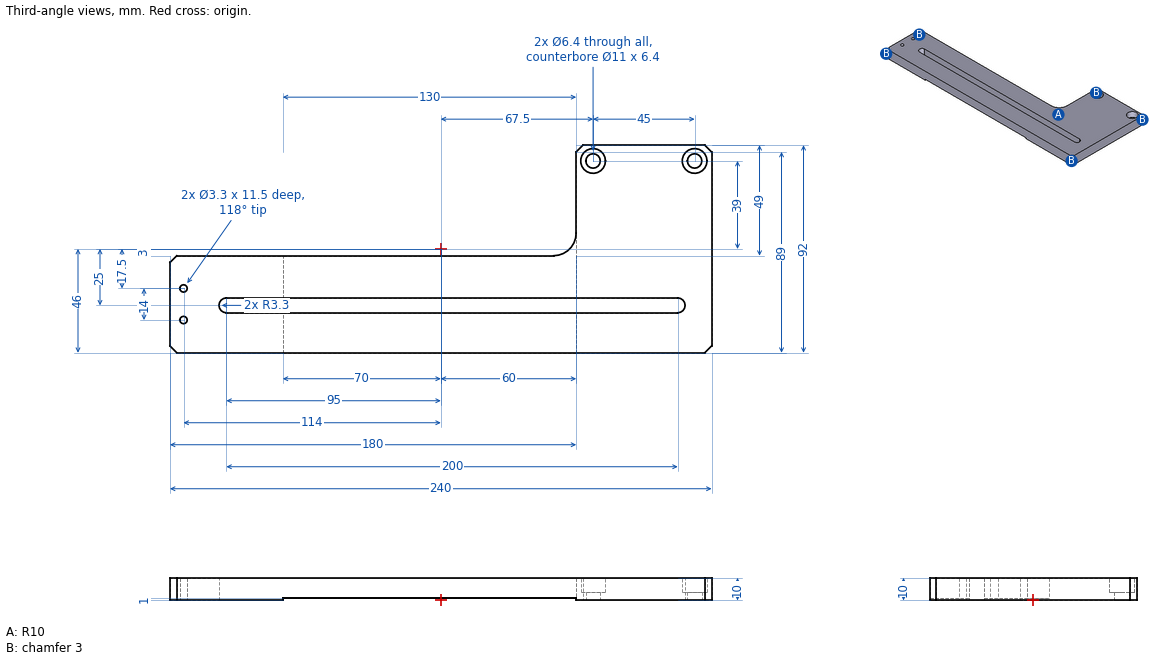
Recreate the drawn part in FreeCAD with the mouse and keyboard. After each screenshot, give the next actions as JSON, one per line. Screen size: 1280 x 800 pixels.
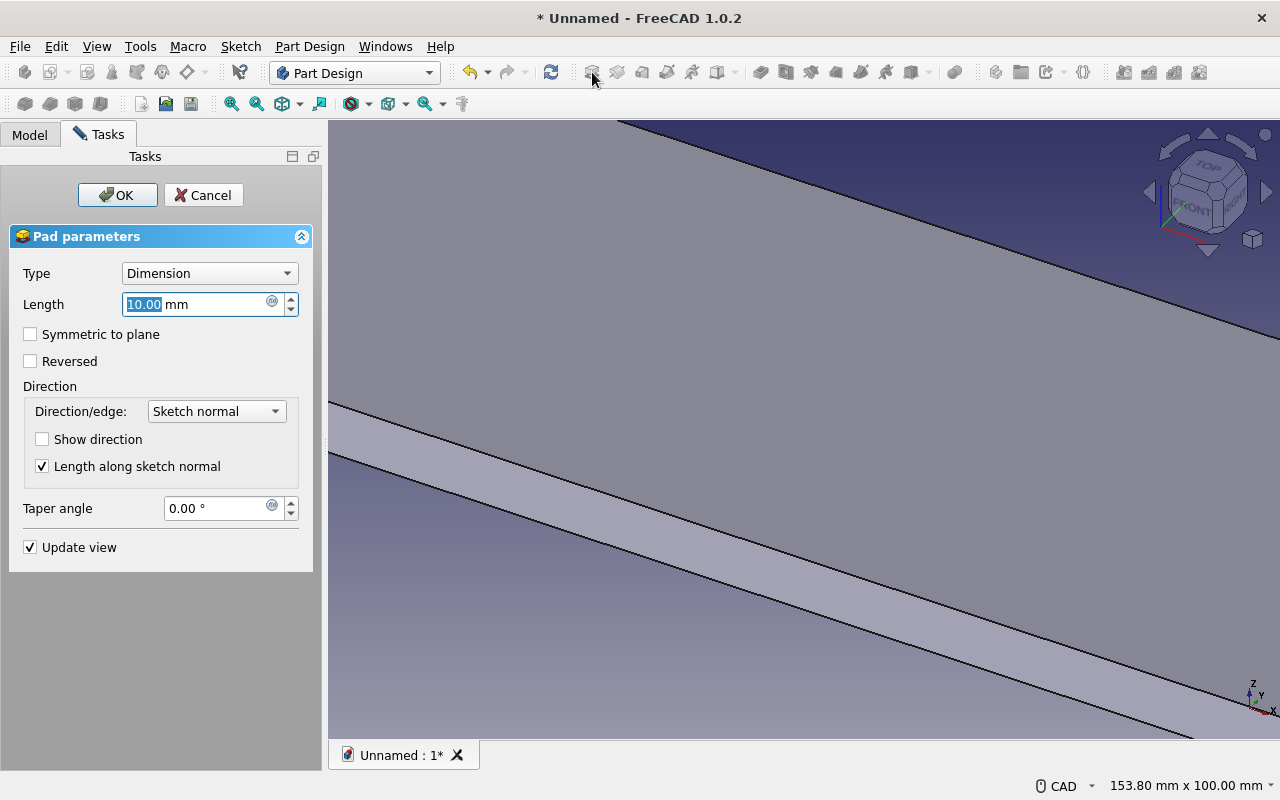
{"action": "type", "text": "10"}
{"action": "key", "text": "Tab"}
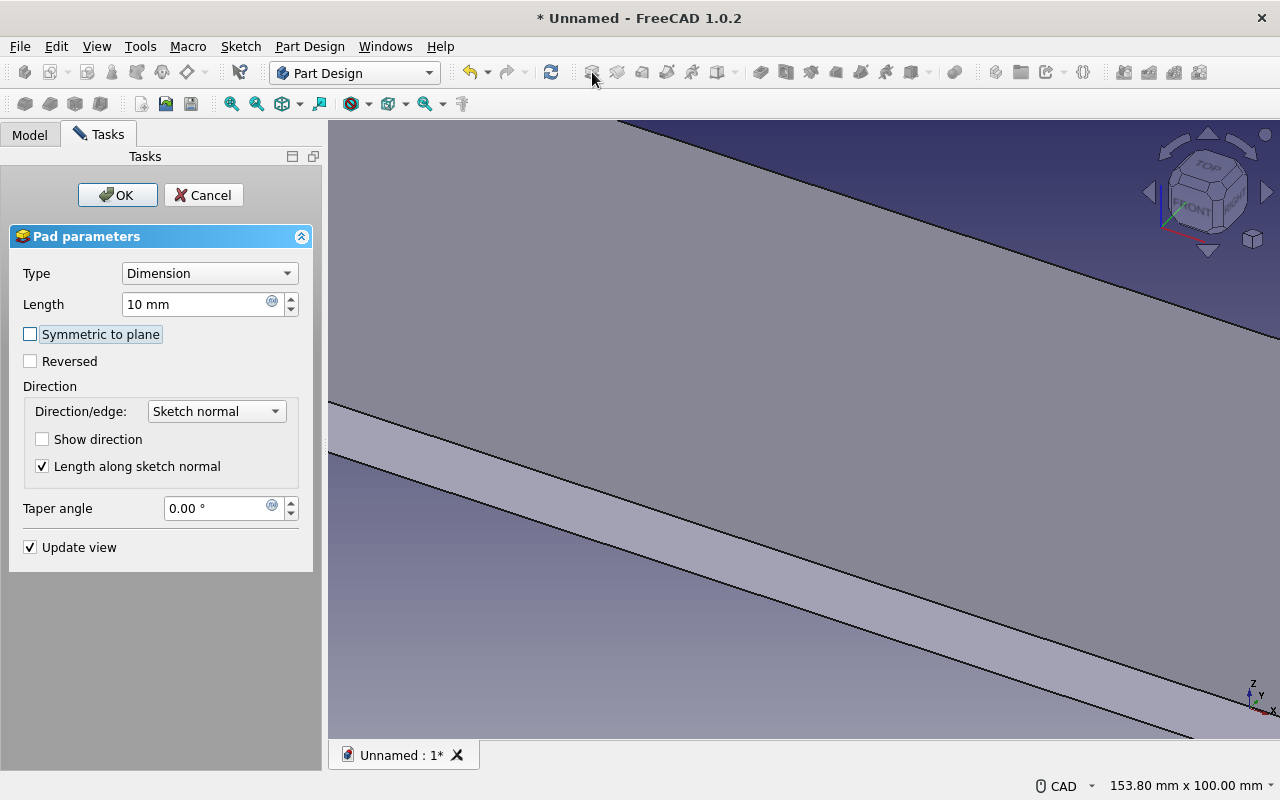
{"action": "left_click", "coordinate": [118, 195]}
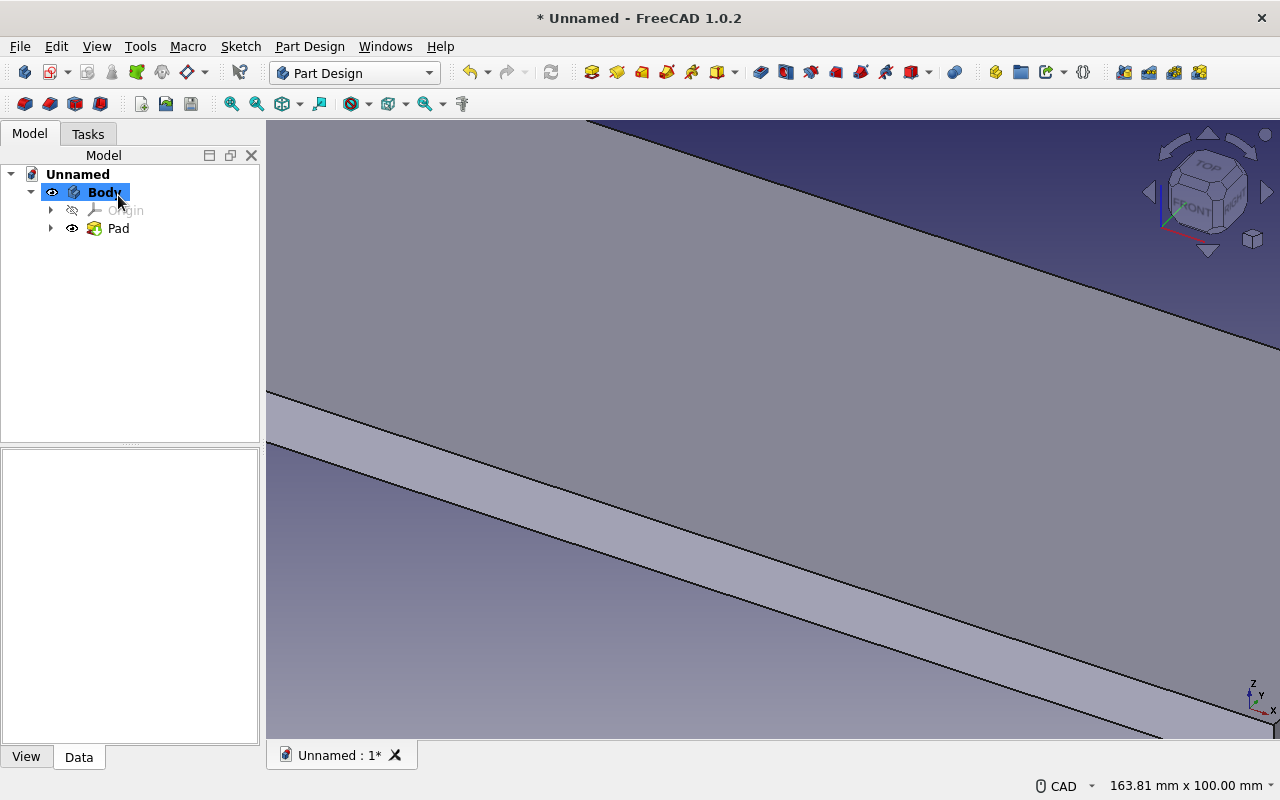
{"action": "key", "text": "v f"}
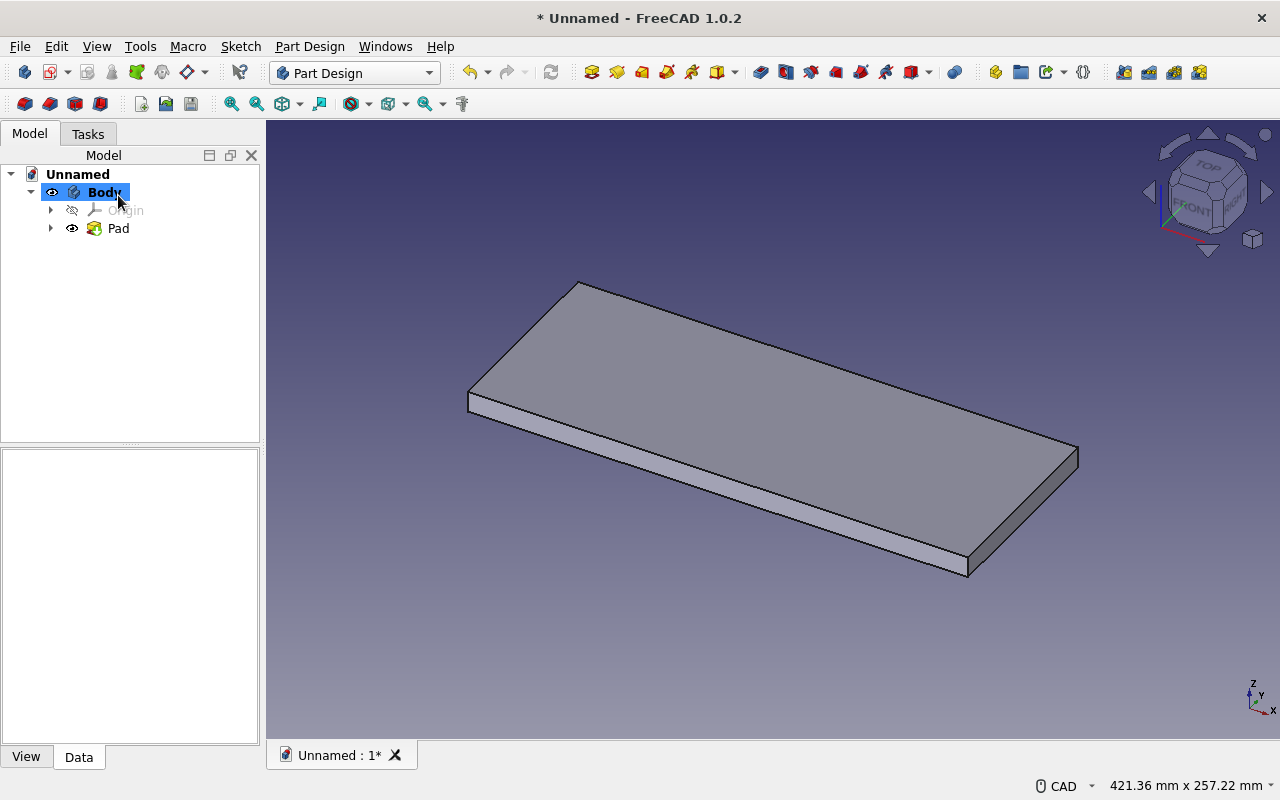
{"action": "left_click", "coordinate": [916, 466]}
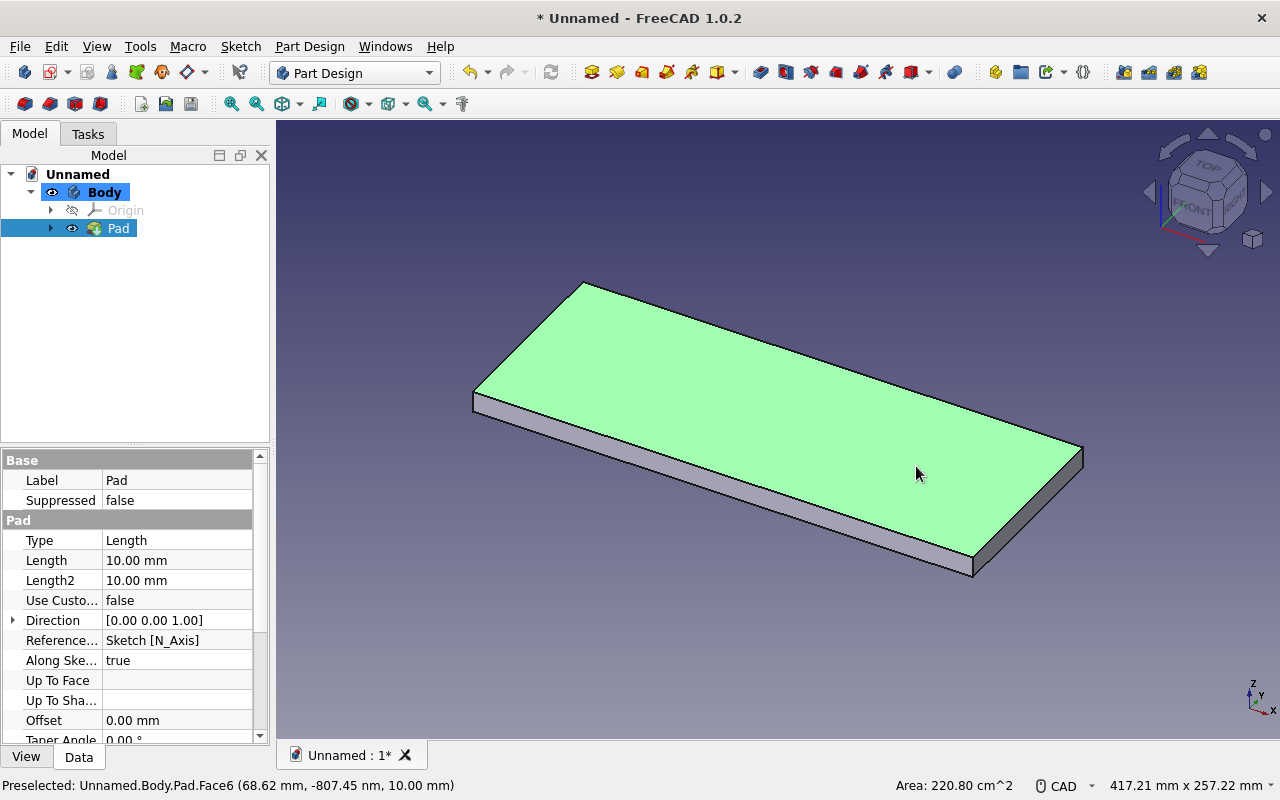
{"action": "left_click", "coordinate": [50, 72]}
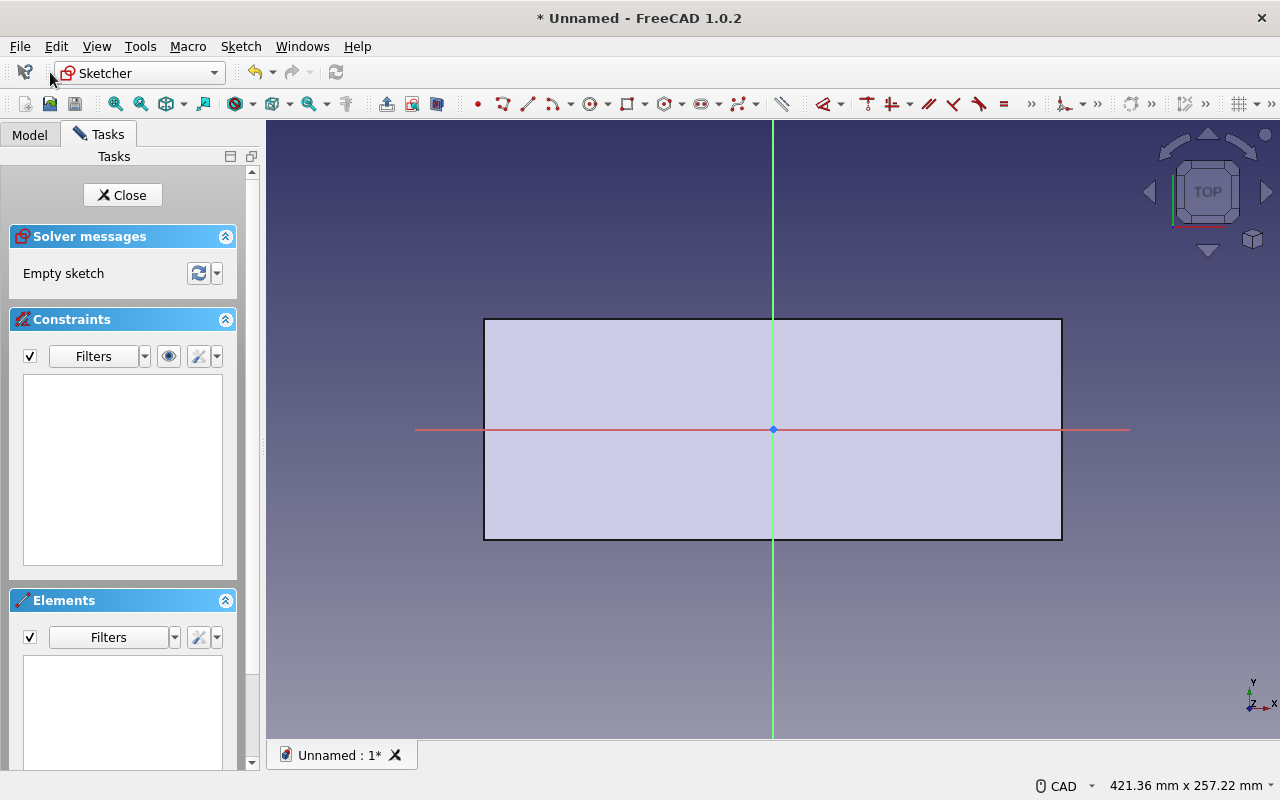
{"action": "key", "text": "g s"}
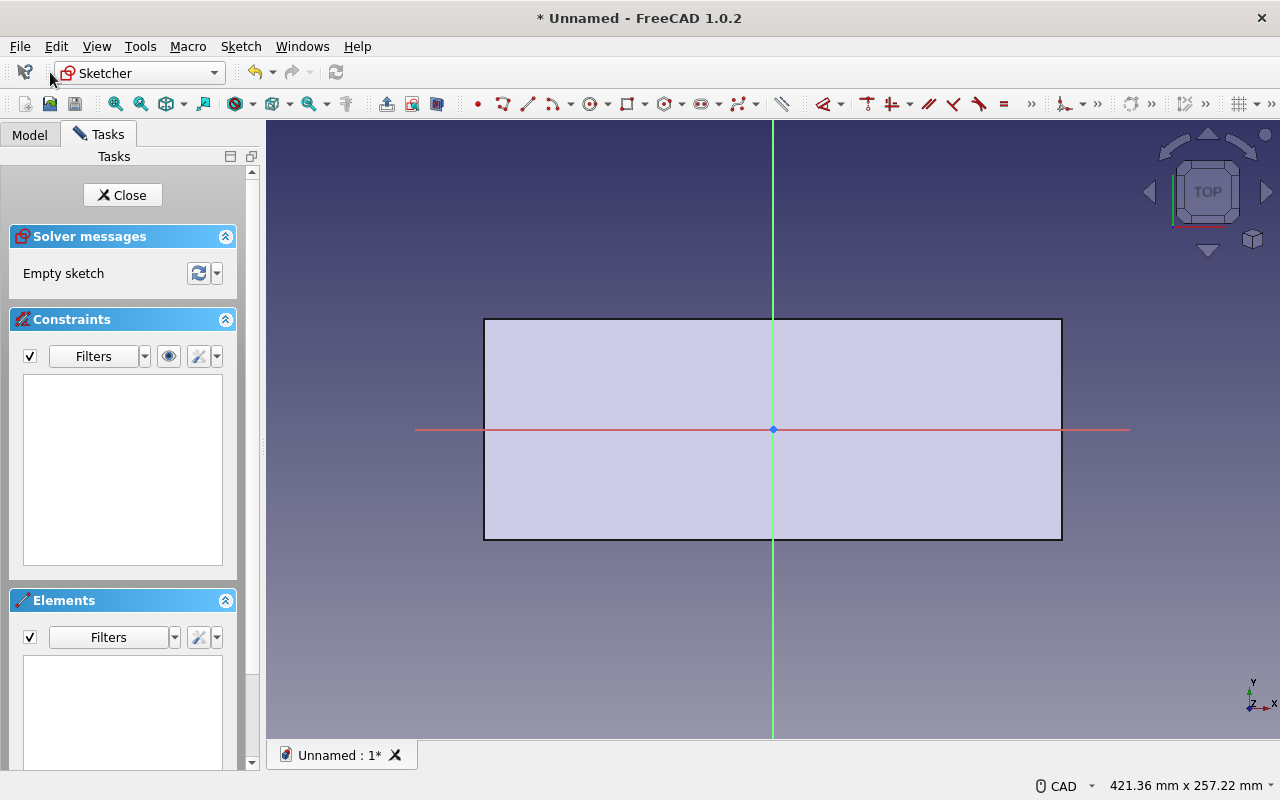
{"action": "scroll", "coordinate": [544, 490], "scroll_direction": "up", "scroll_amount": 6}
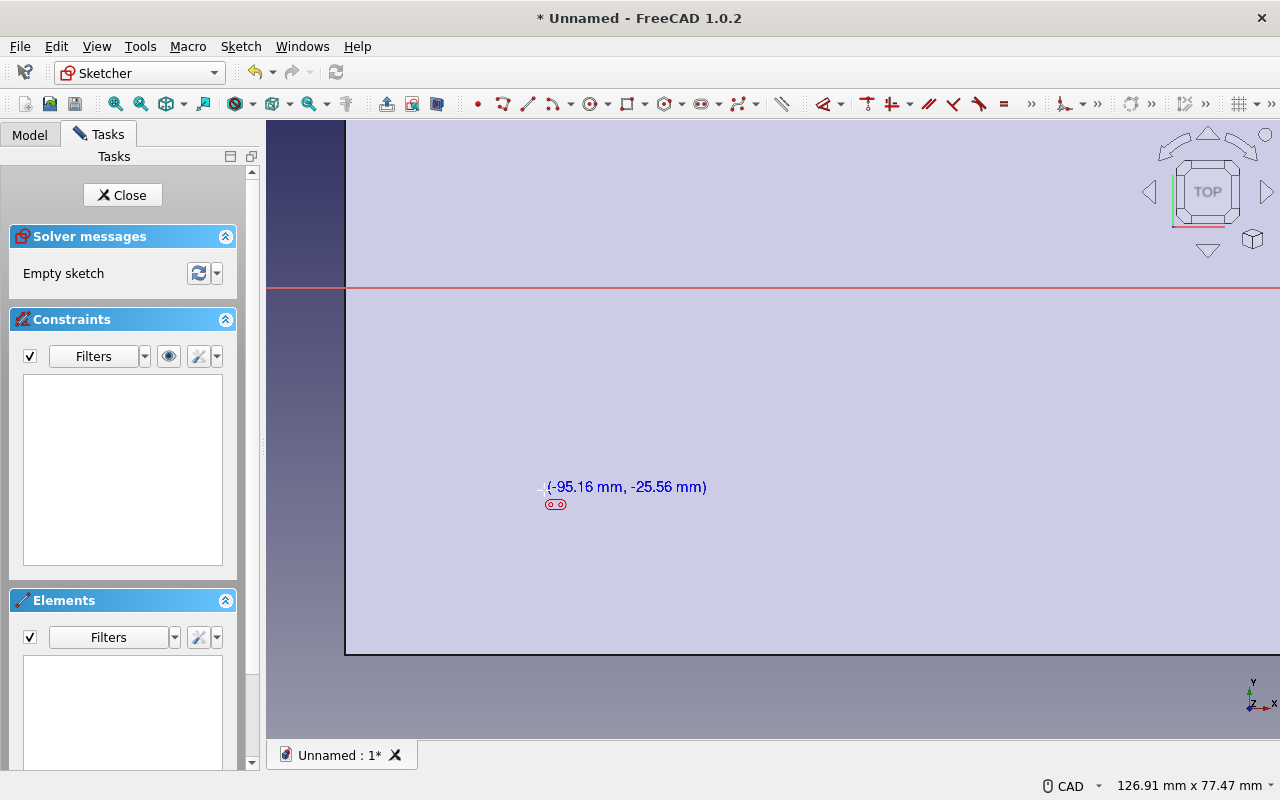
{"action": "left_click", "coordinate": [545, 487]}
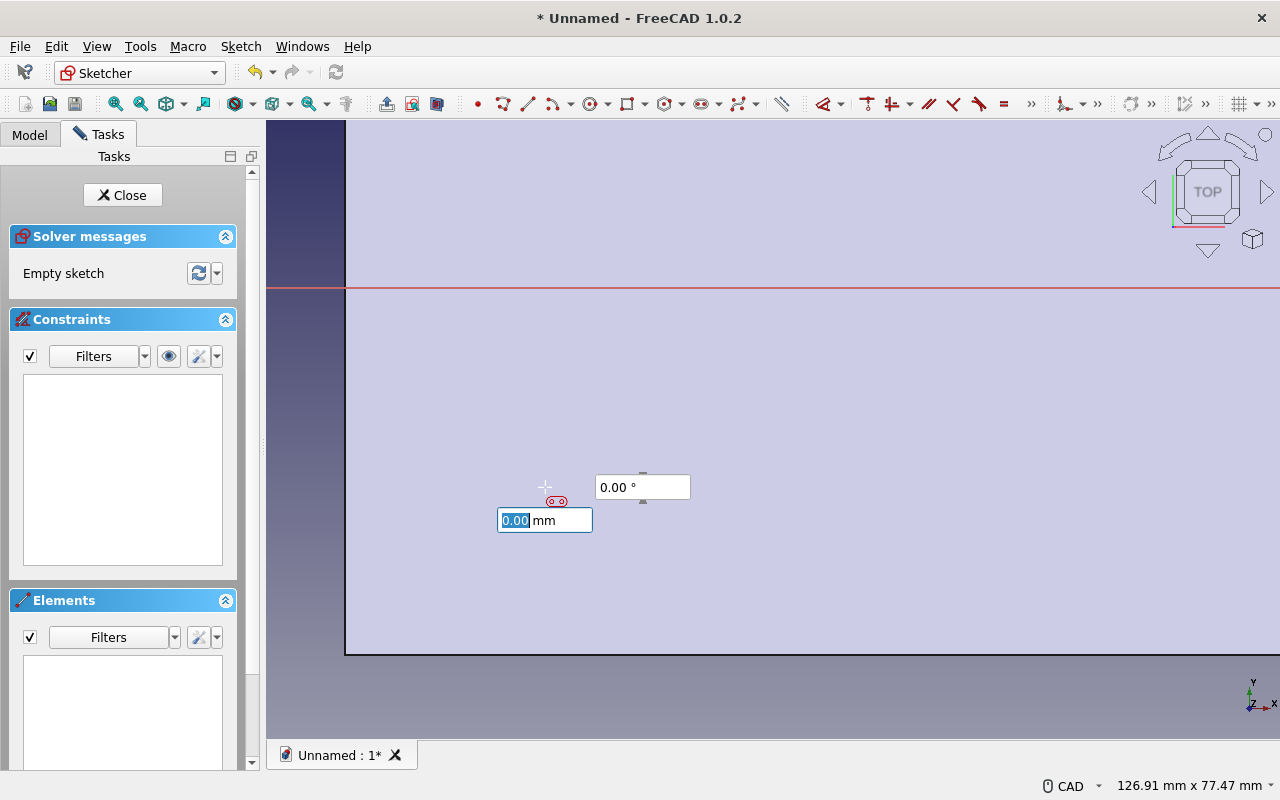
{"action": "scroll", "coordinate": [333, 446], "scroll_direction": "down", "scroll_amount": 5}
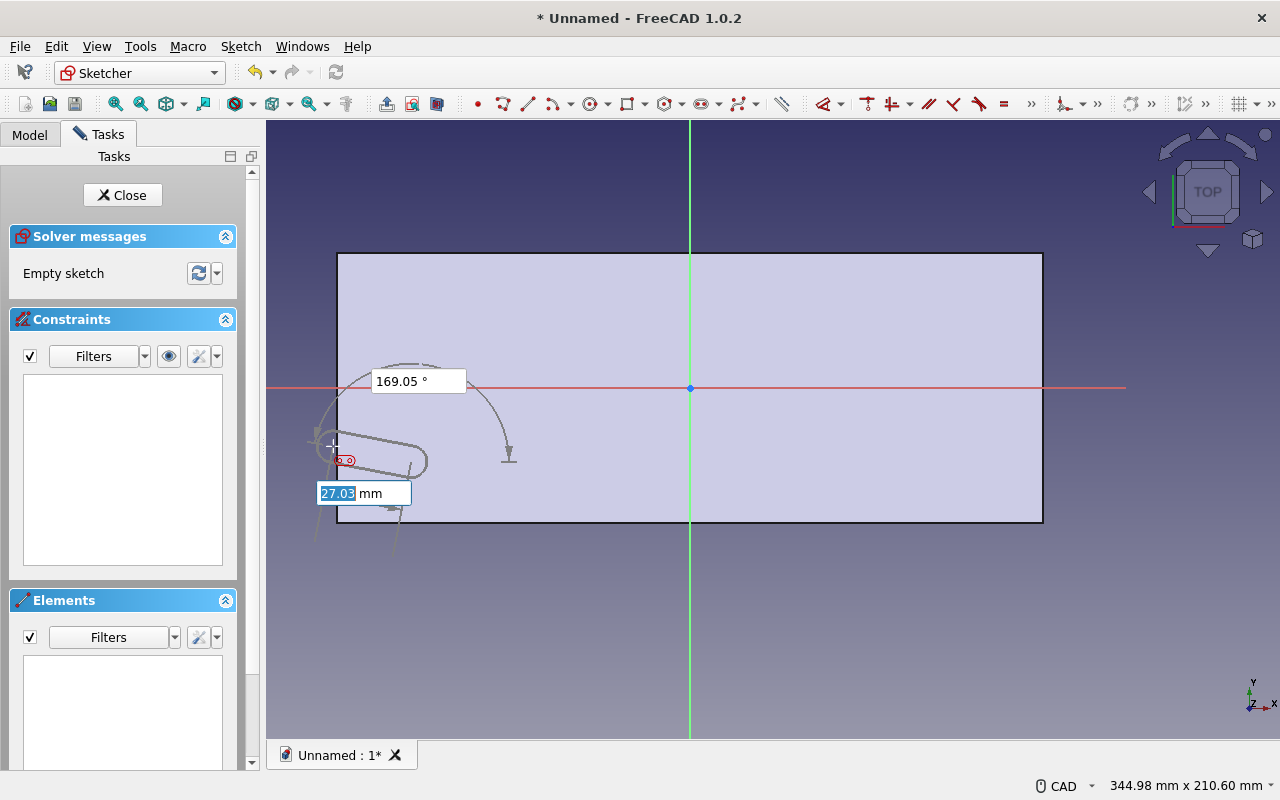
{"action": "left_click", "coordinate": [999, 461]}